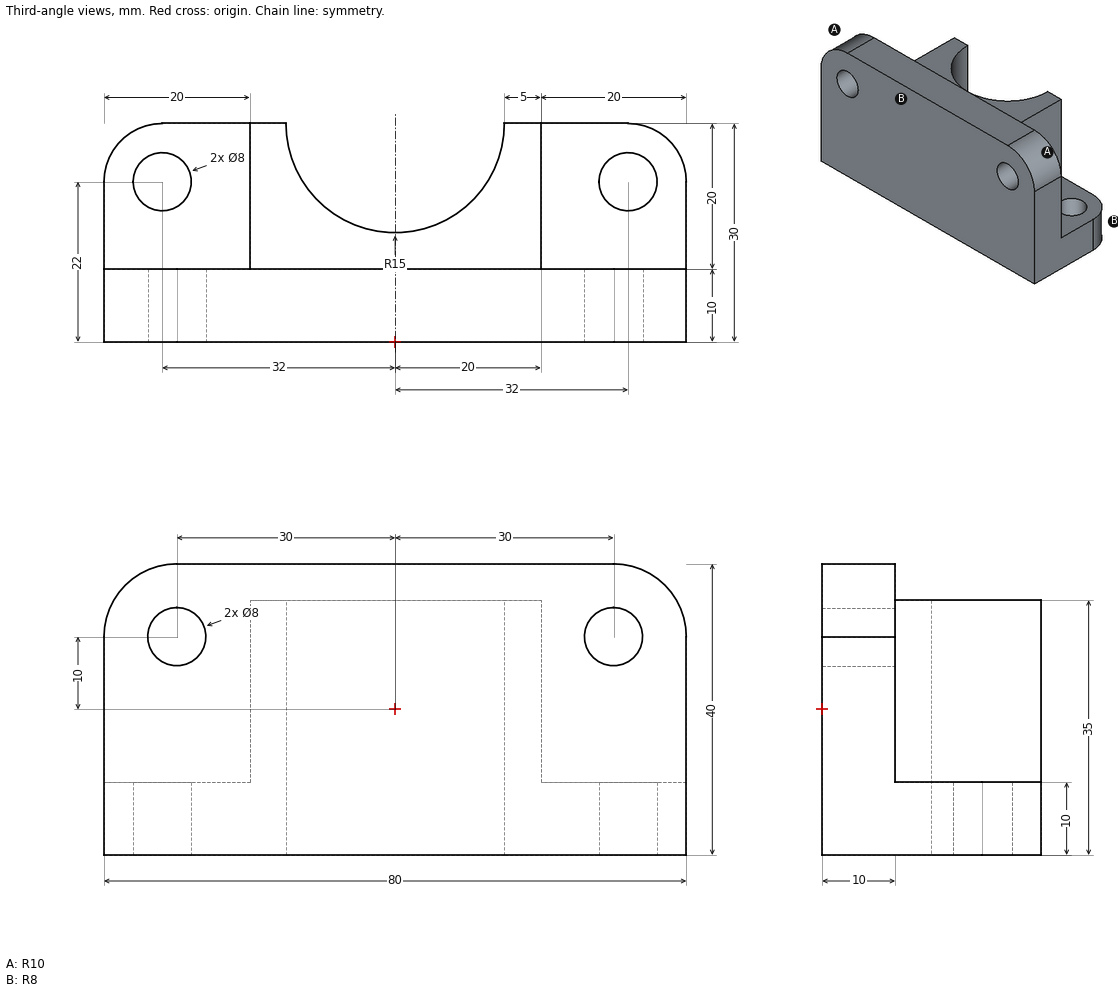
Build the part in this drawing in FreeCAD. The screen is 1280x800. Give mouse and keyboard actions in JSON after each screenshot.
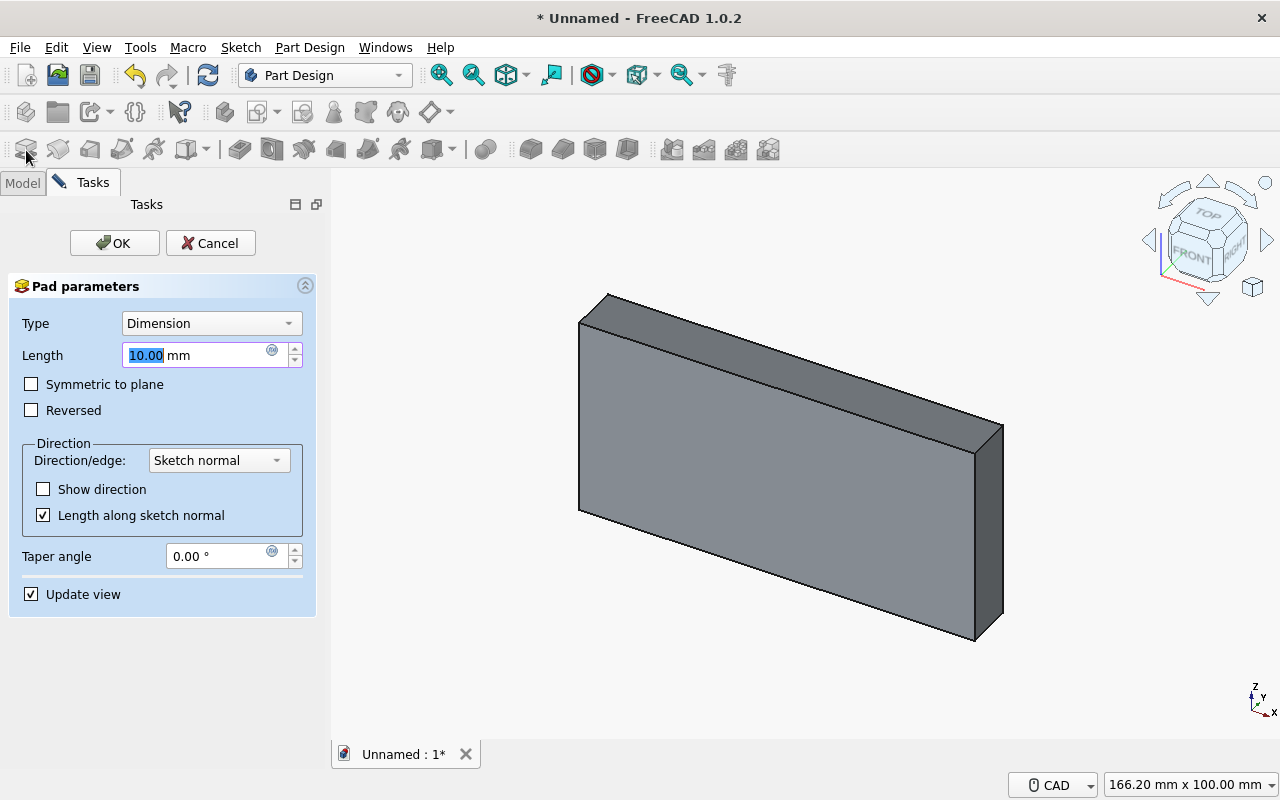
{"action": "type", "text": "10"}
{"action": "key", "text": "Tab"}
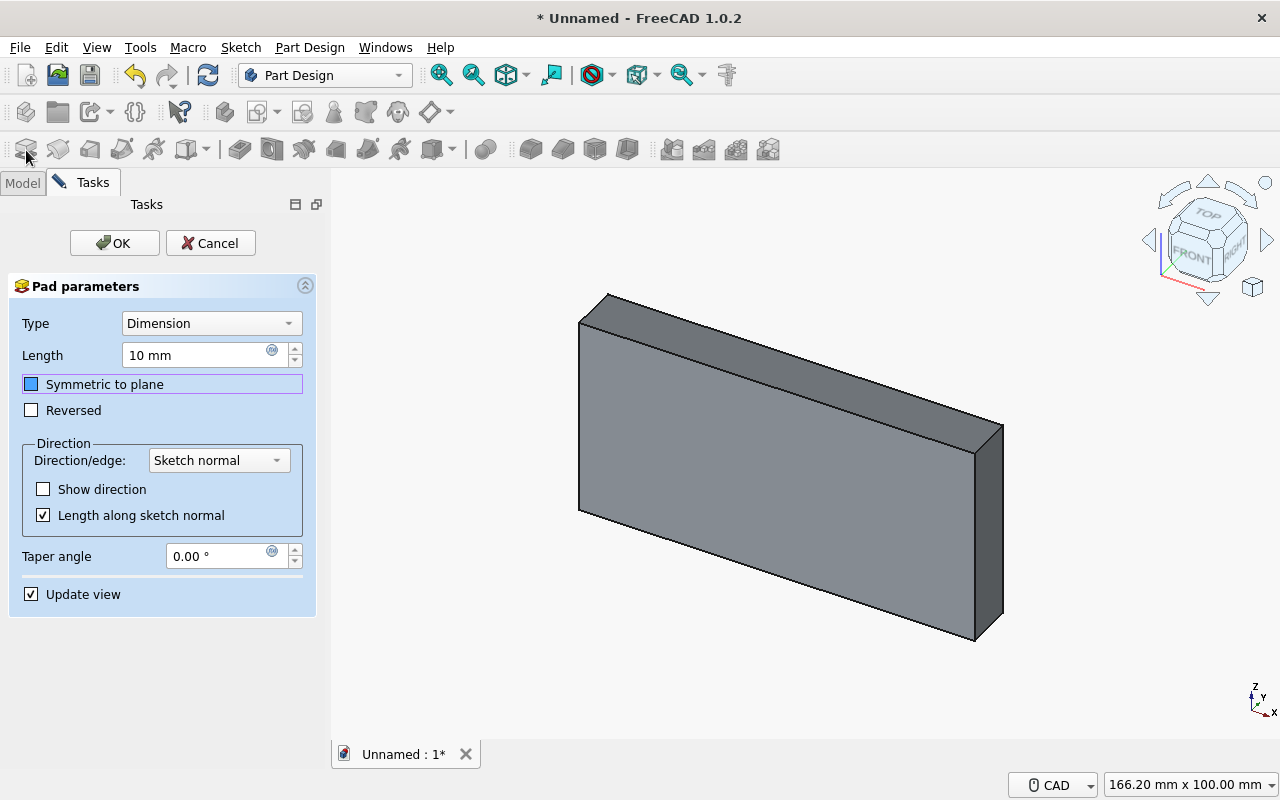
{"action": "left_click", "coordinate": [30, 410]}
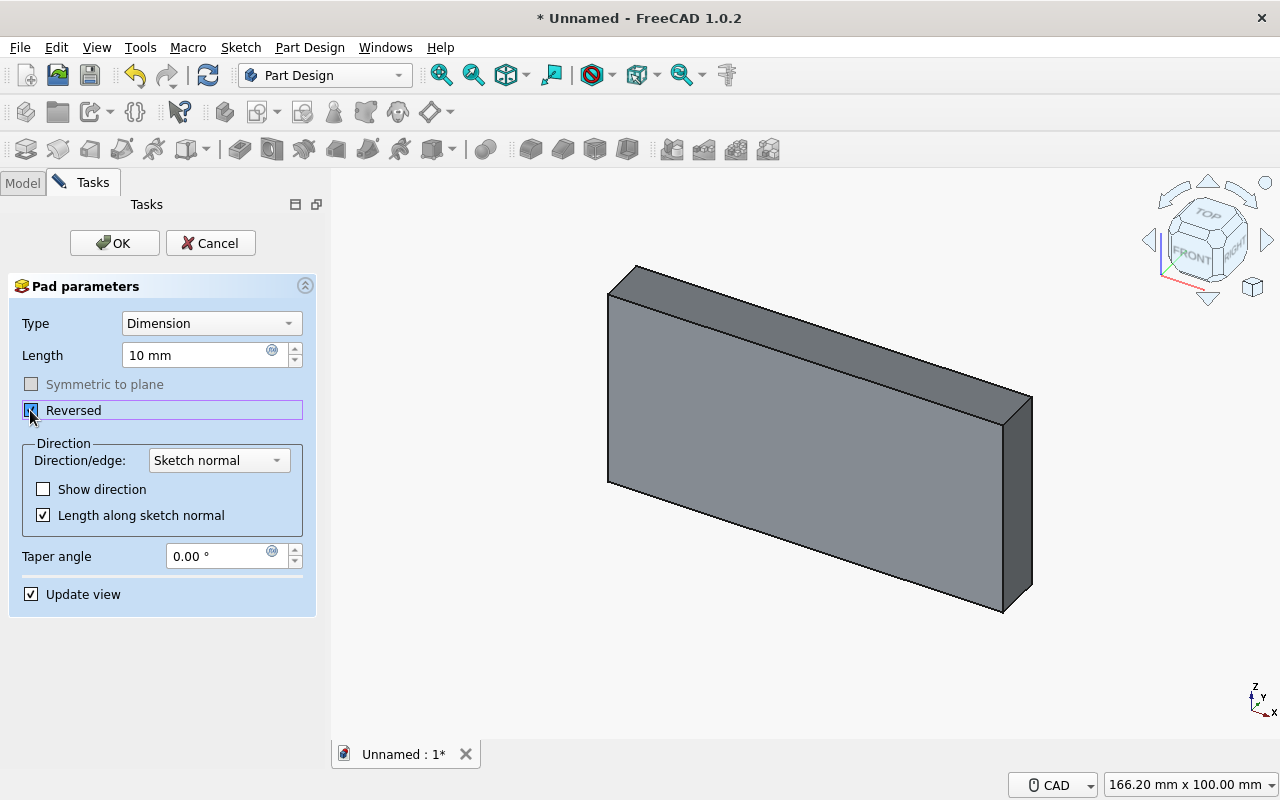
{"action": "left_click", "coordinate": [115, 243]}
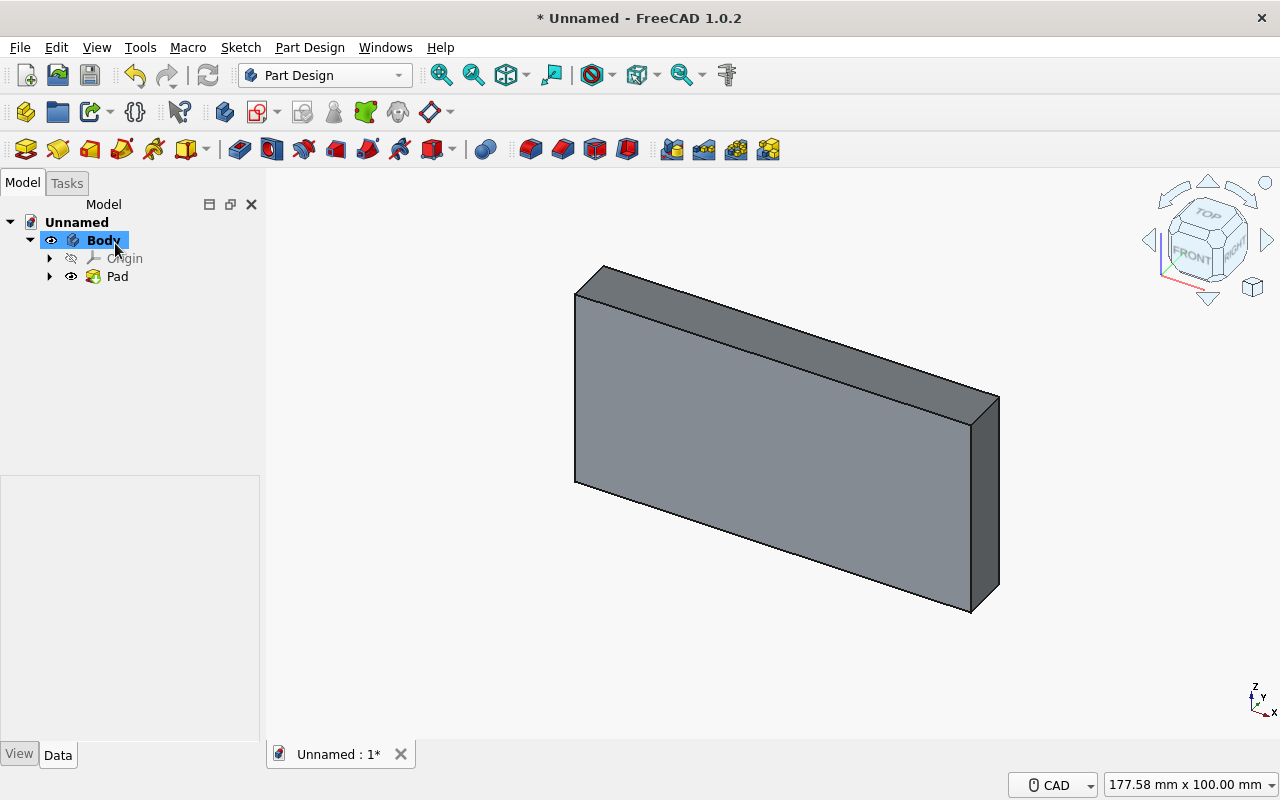
{"action": "left_click", "coordinate": [985, 410]}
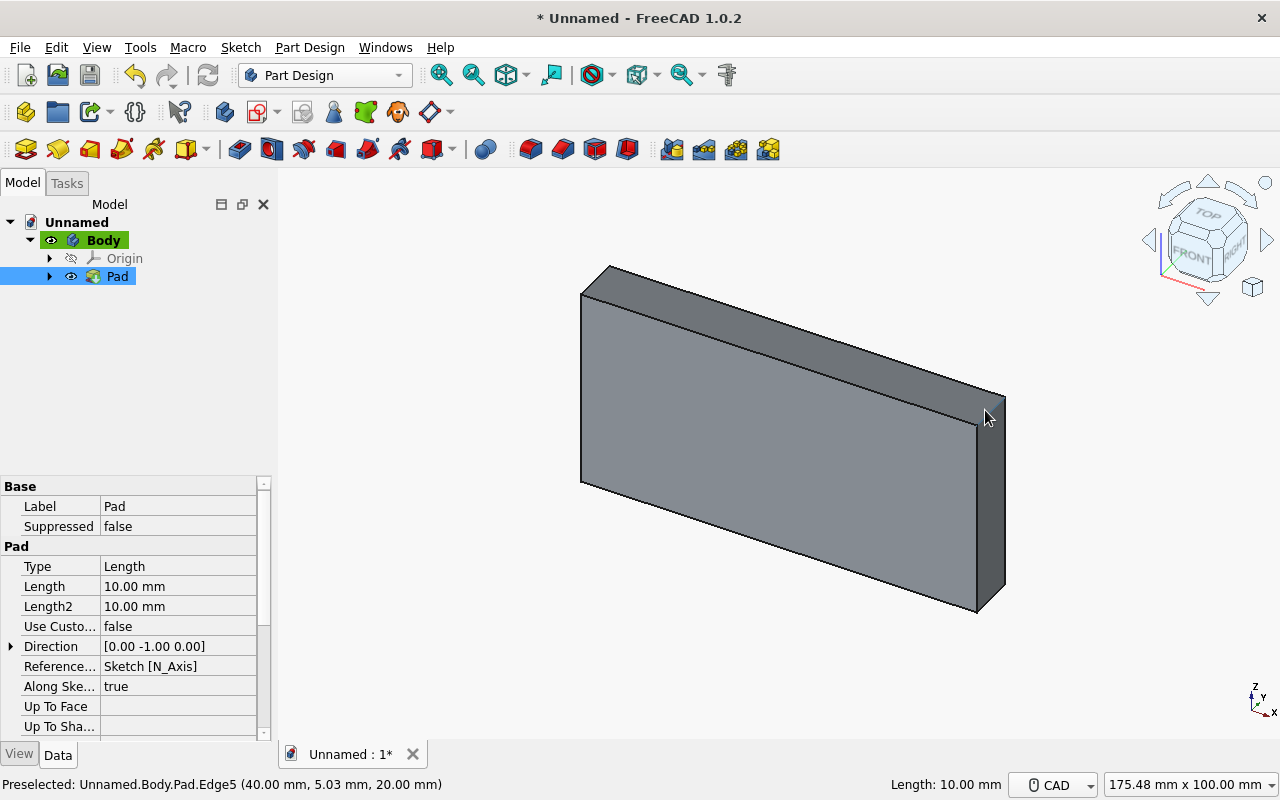
{"action": "key", "text": "0"}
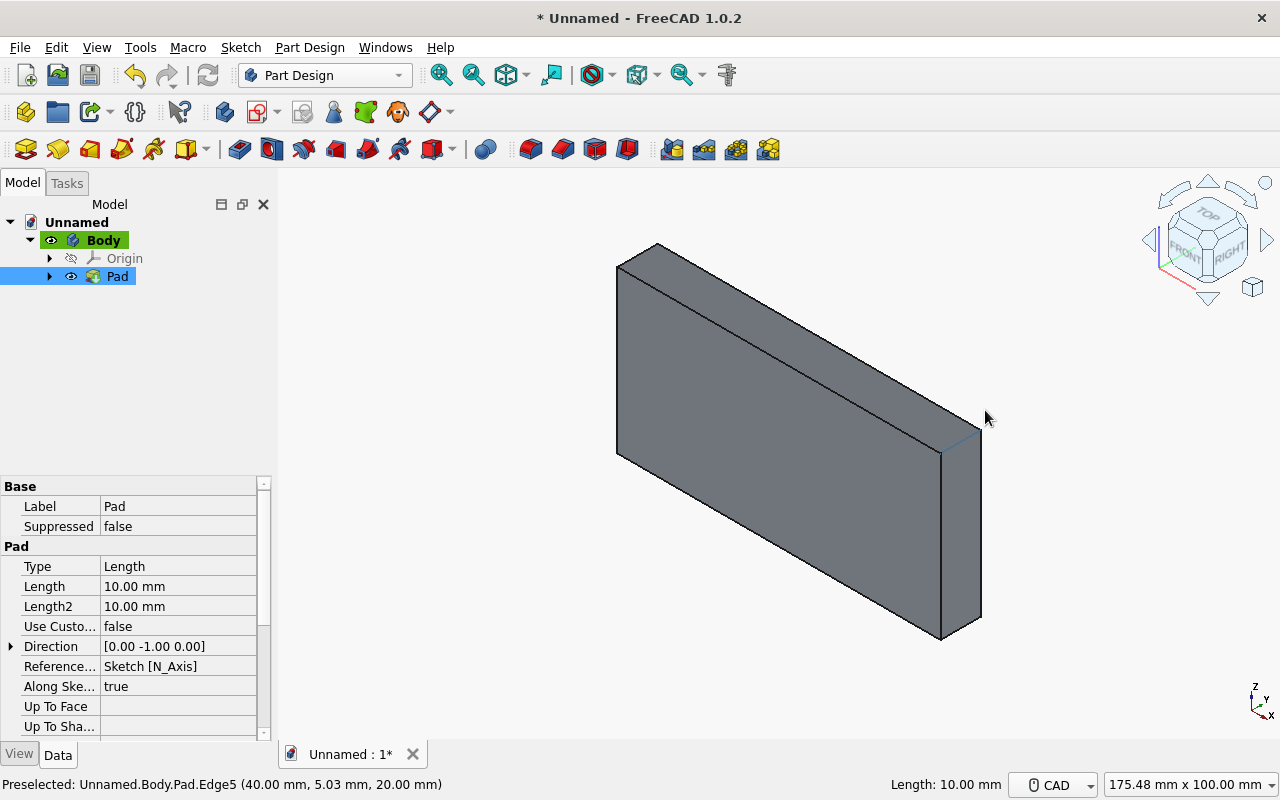
{"action": "key", "text": "2"}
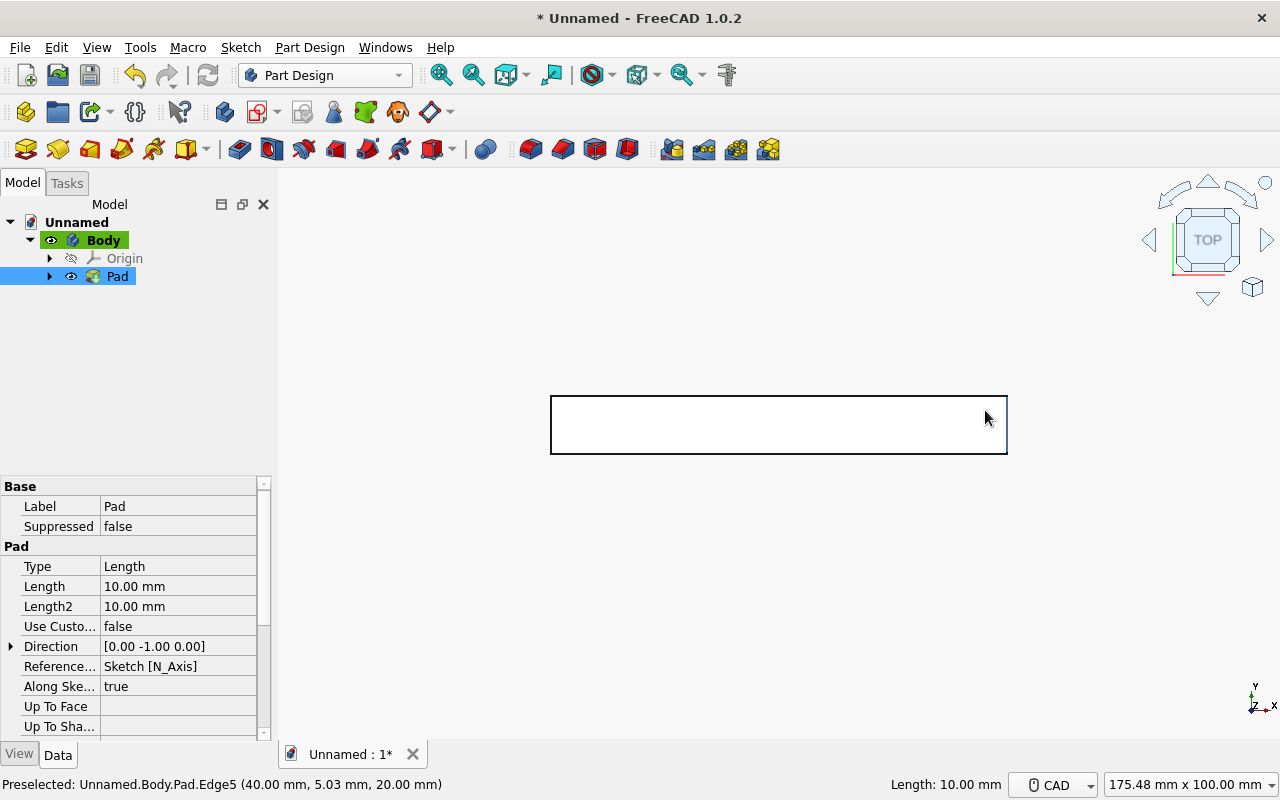
{"action": "left_click", "coordinate": [551, 424], "text": "ctrl"}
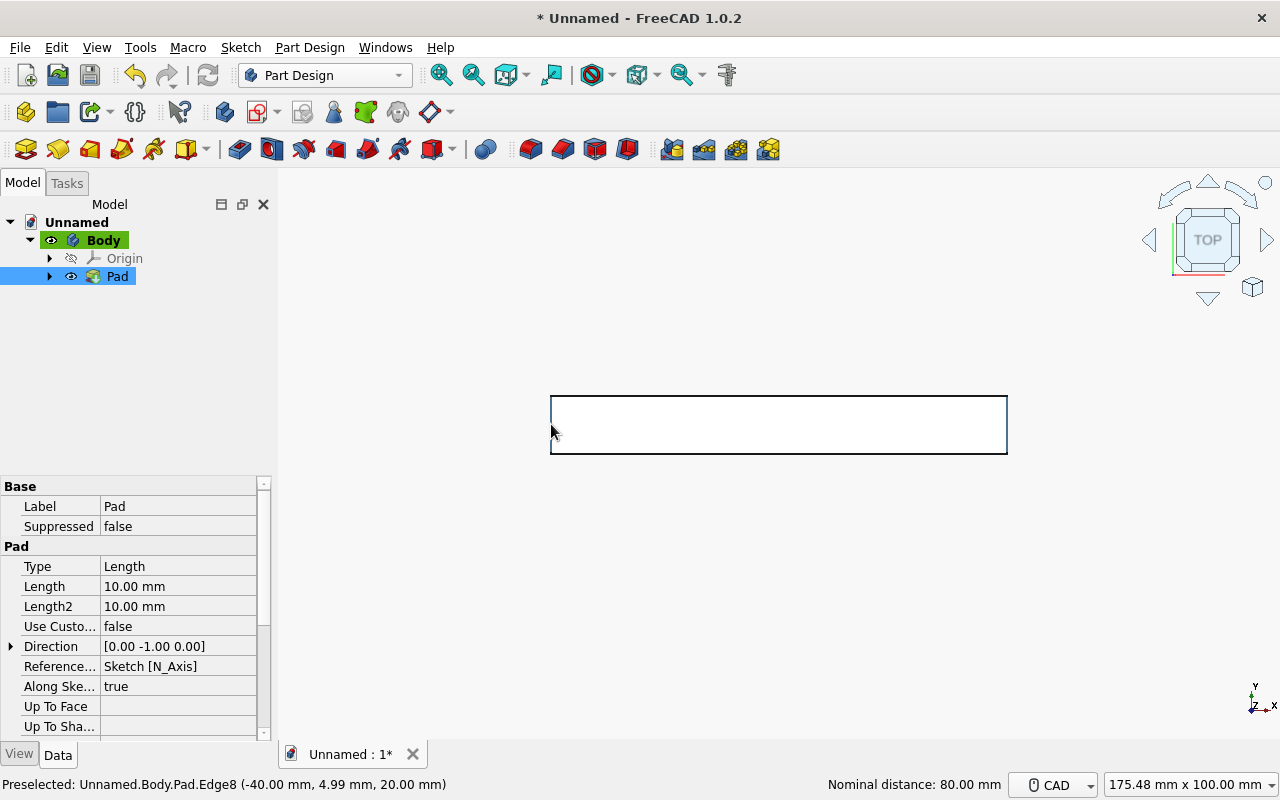
{"action": "left_click", "coordinate": [532, 150]}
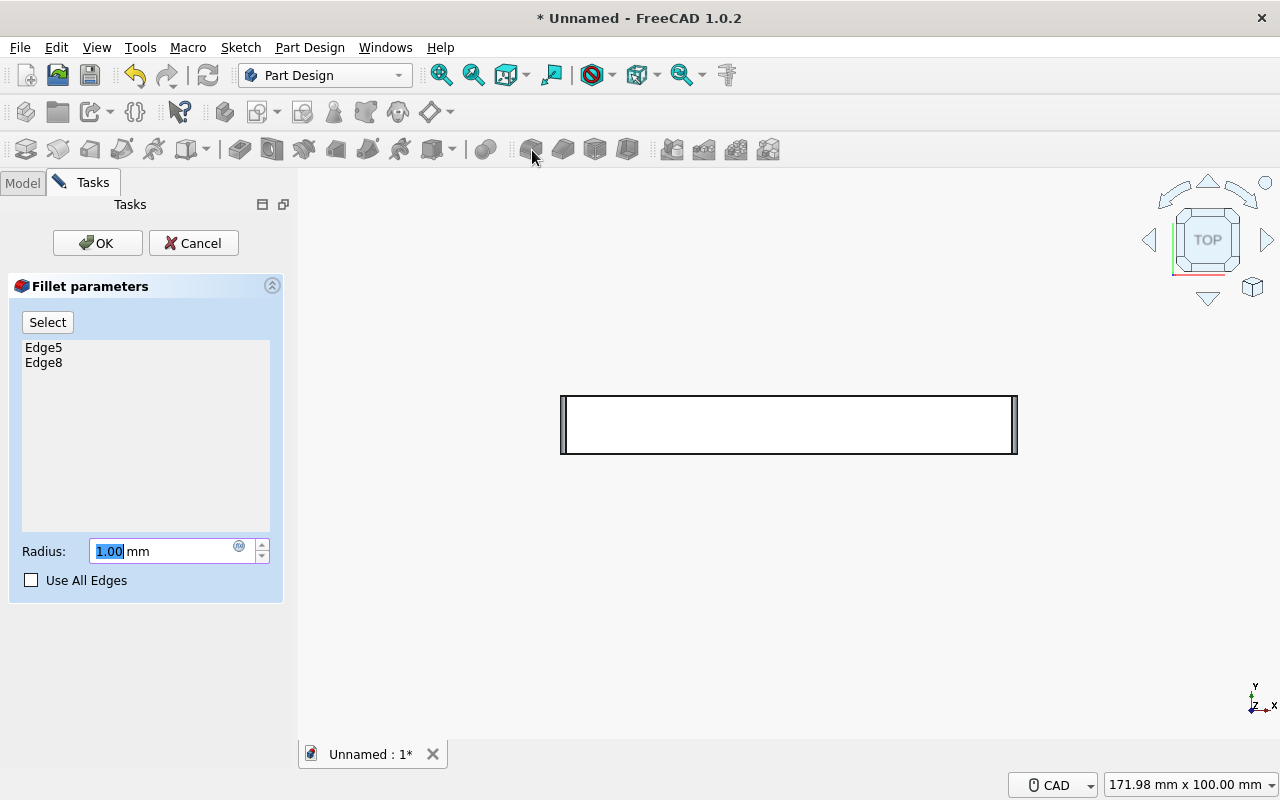
{"action": "type", "text": "10"}
{"action": "key", "text": "Tab"}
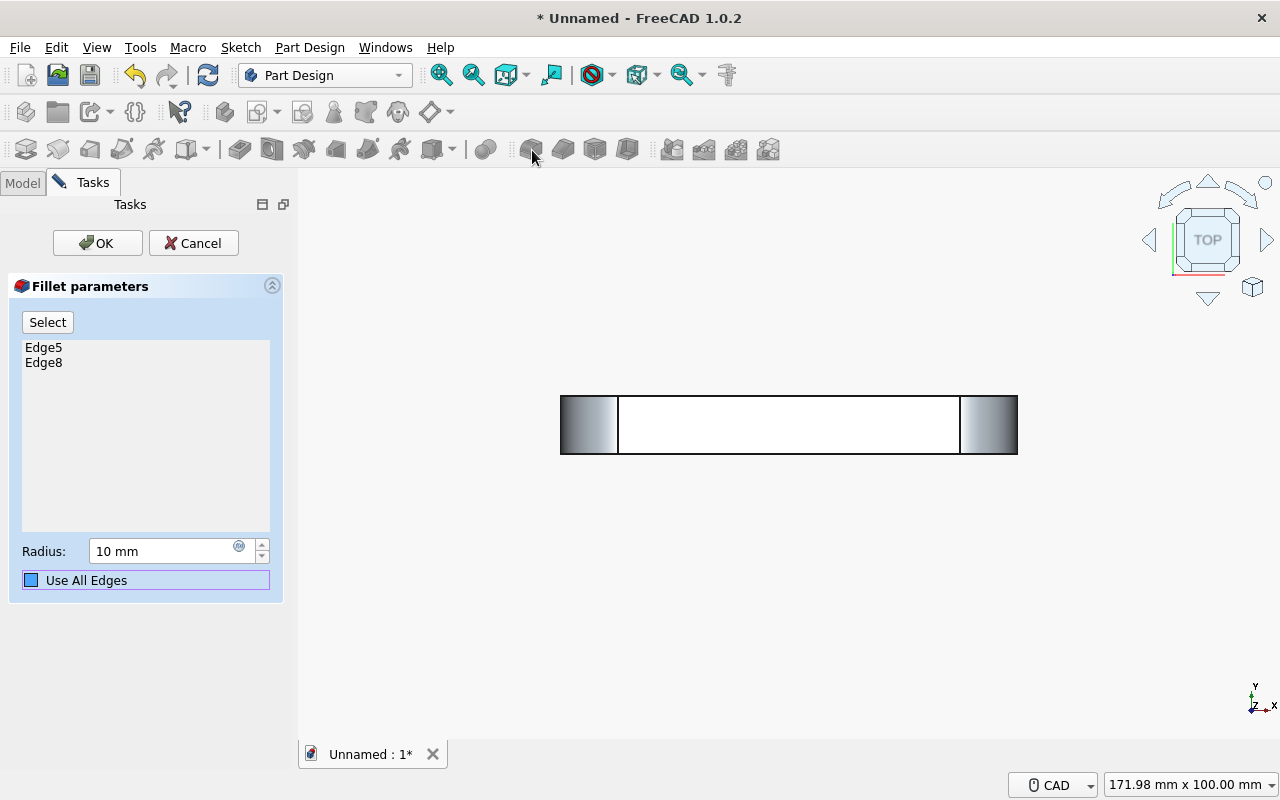
{"action": "left_click", "coordinate": [98, 243]}